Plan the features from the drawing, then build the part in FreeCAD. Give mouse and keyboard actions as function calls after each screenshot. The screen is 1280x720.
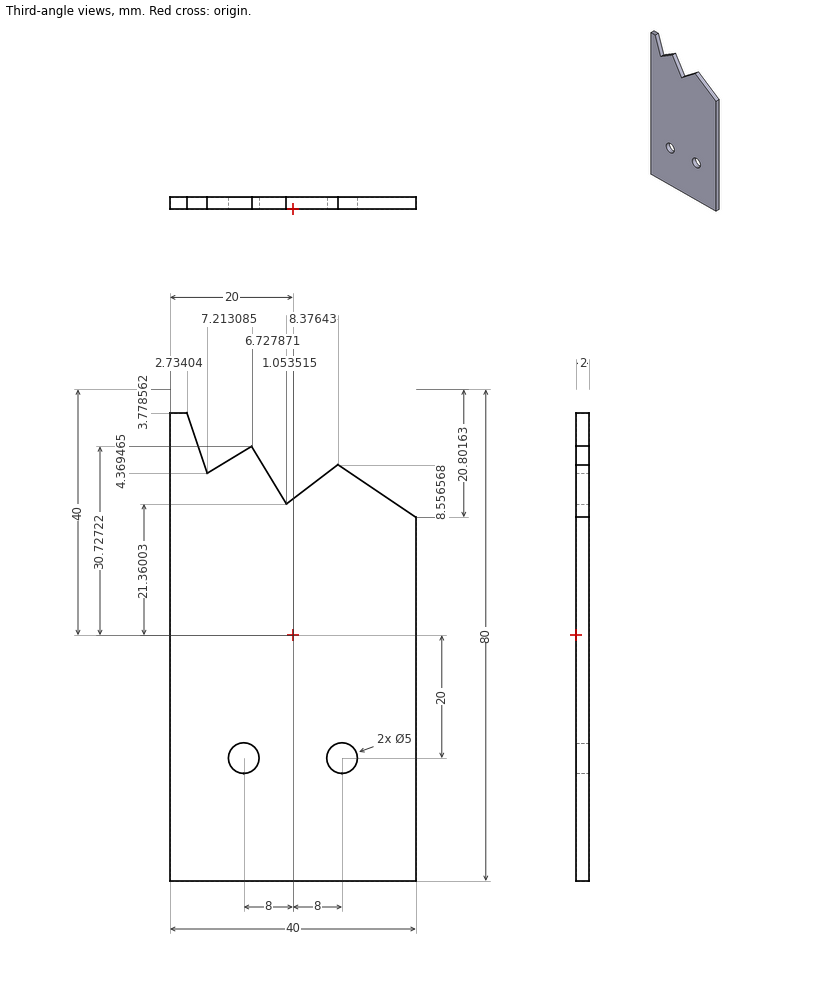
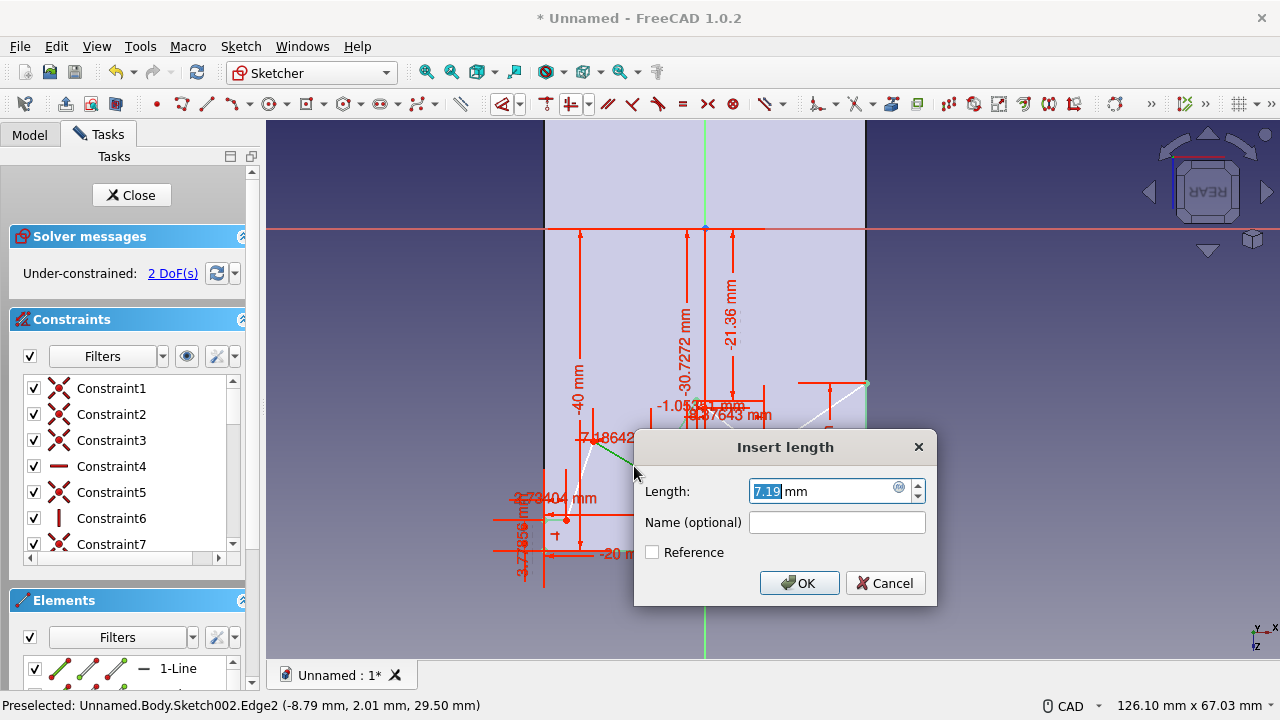
text(7.213085)
key(Return)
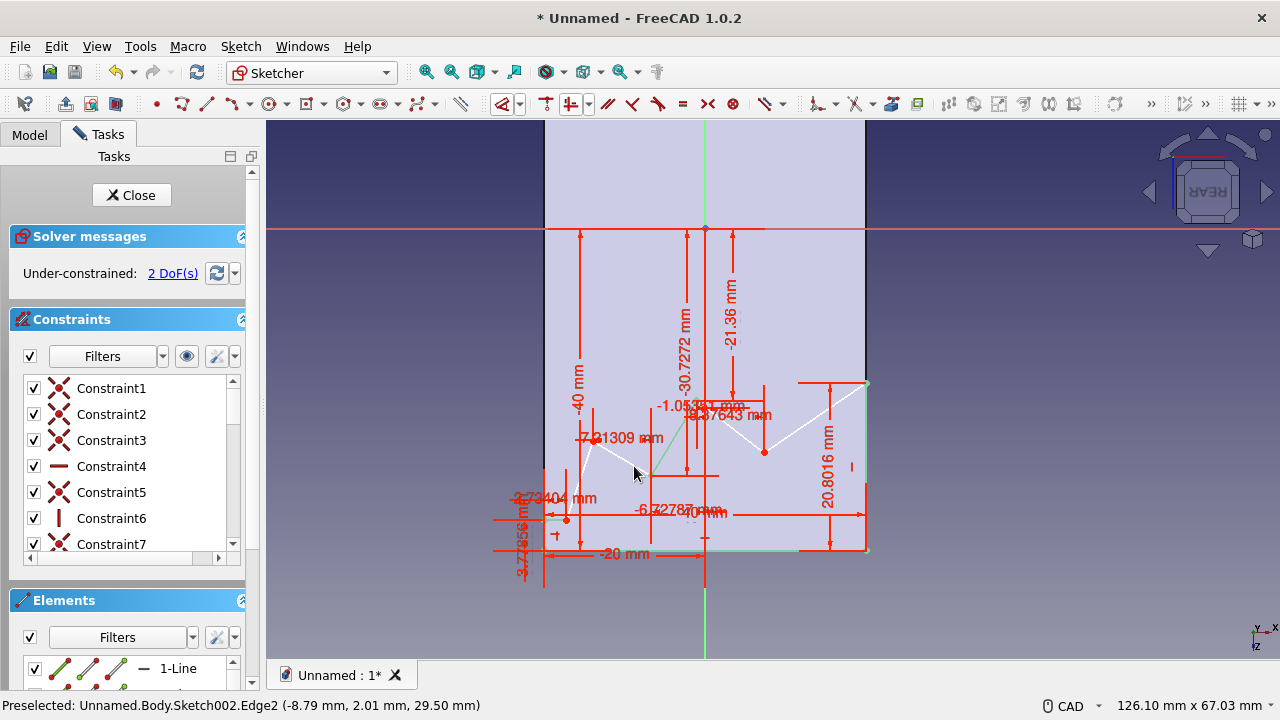
click(634, 466)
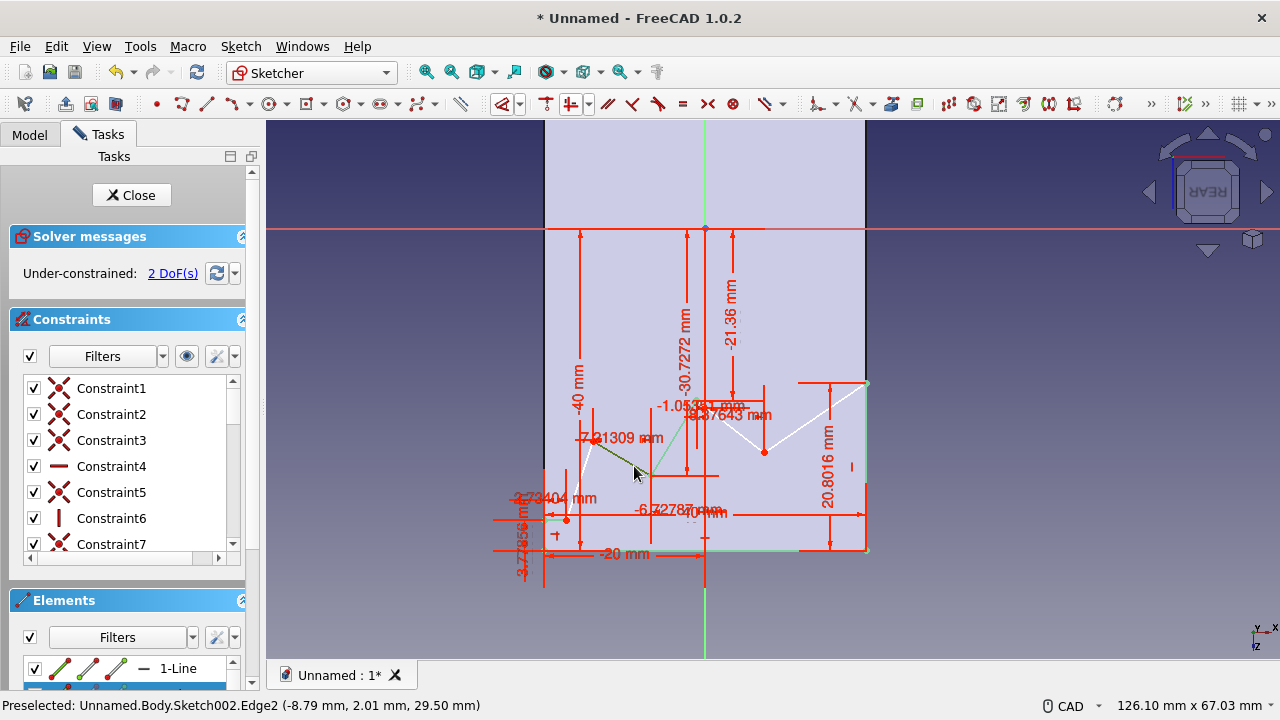
key(i)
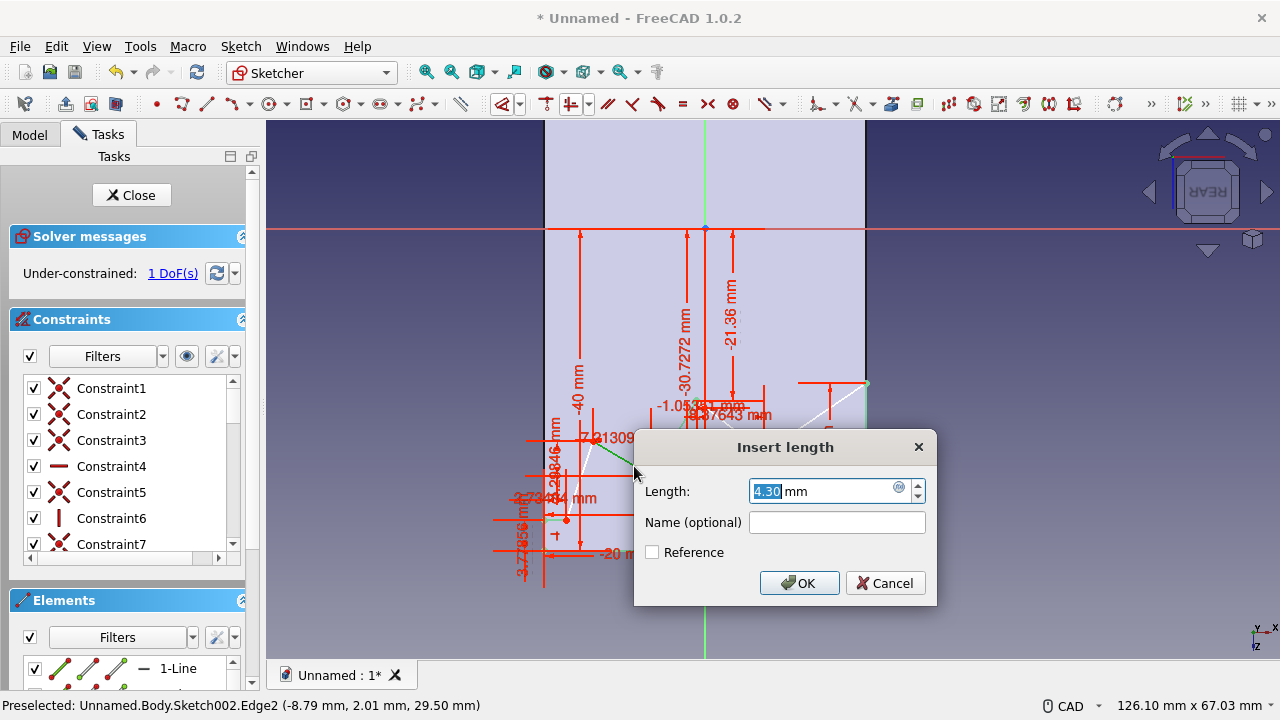
text(4.369465)
key(Return)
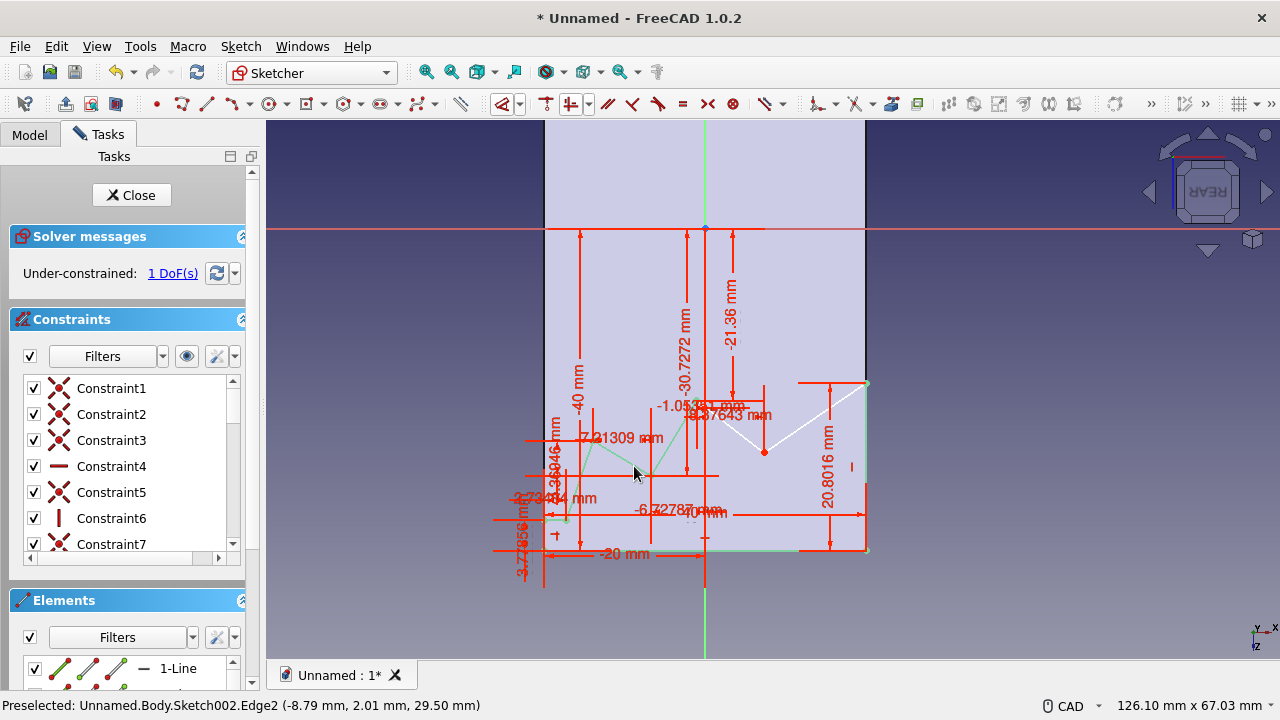
click(835, 404)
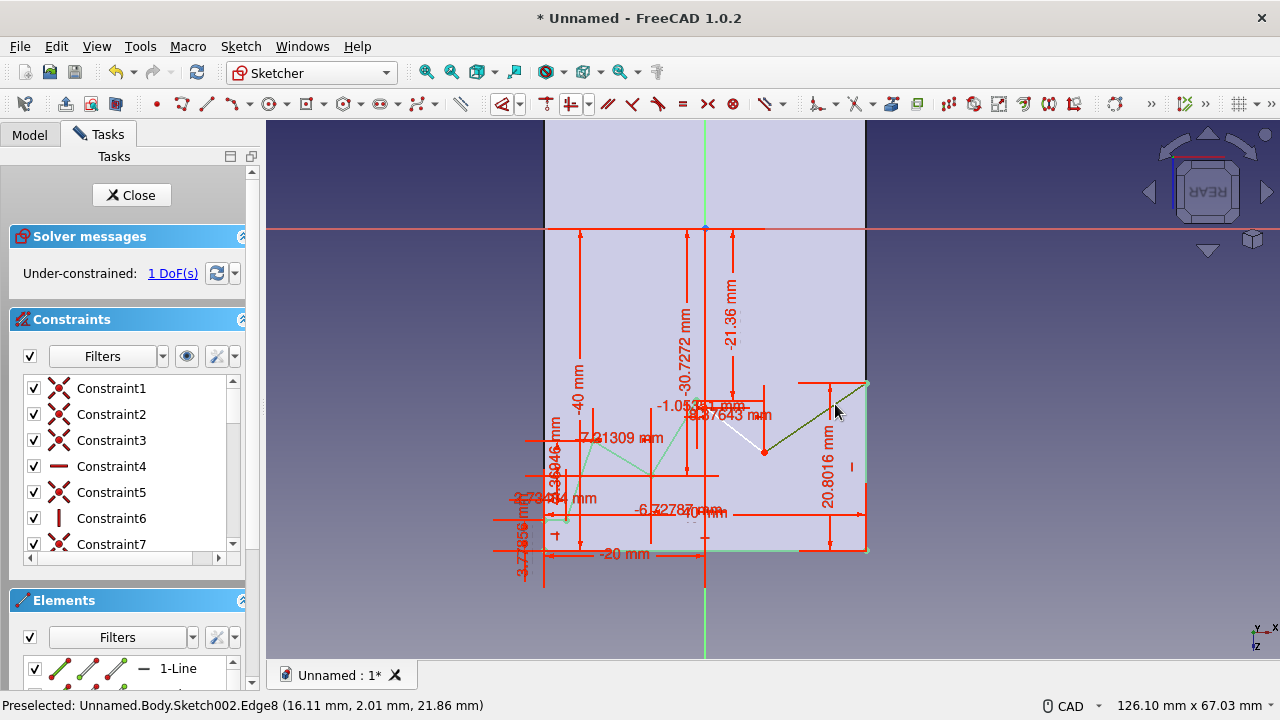
key(i)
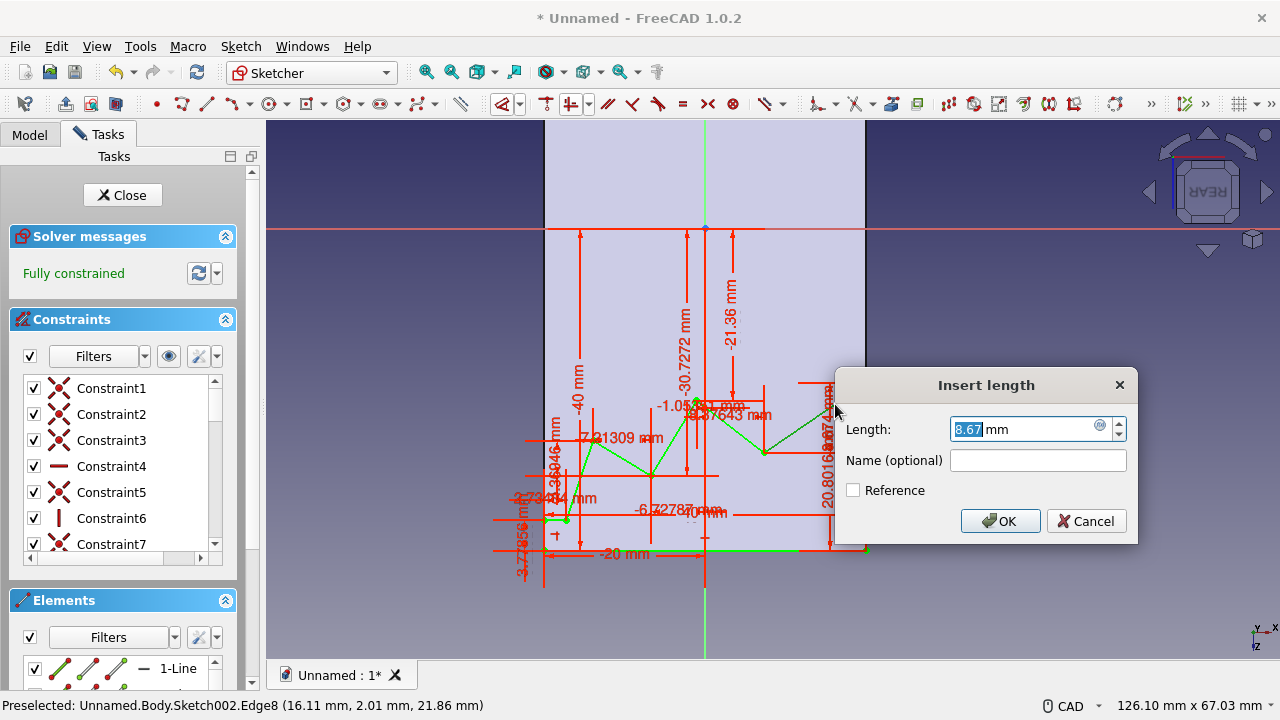
text(8.556568)
key(Return)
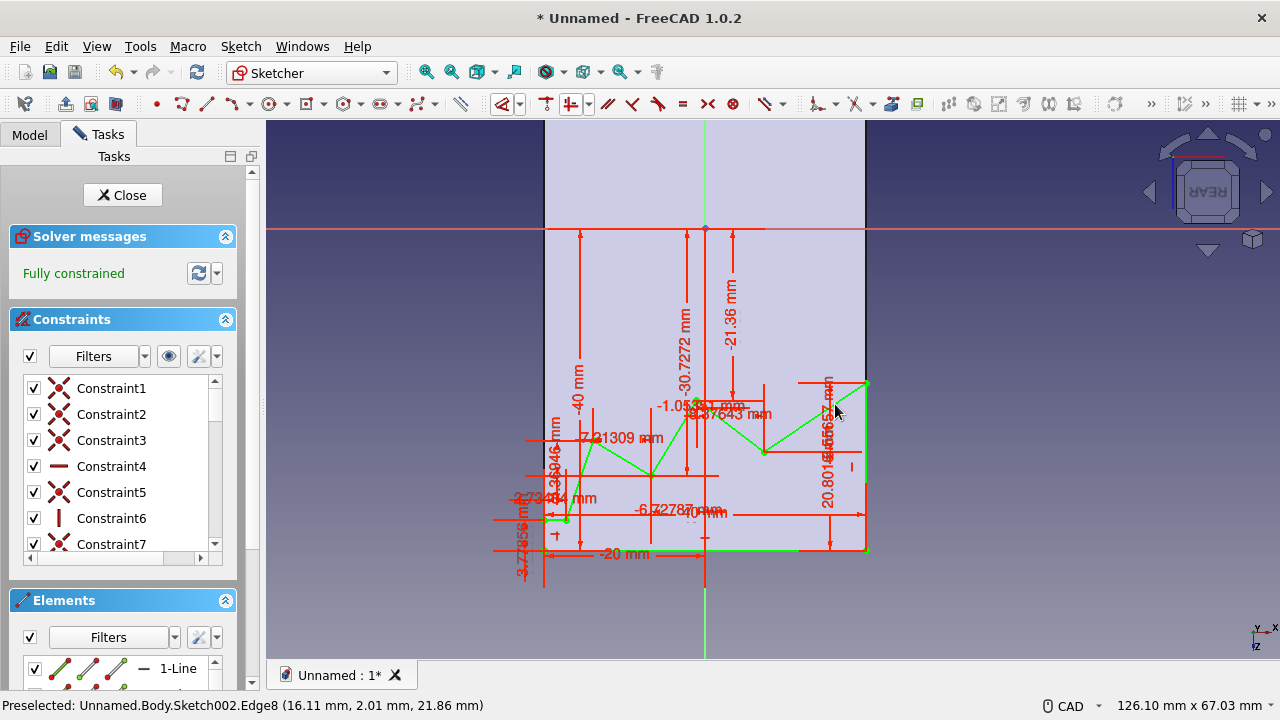
click(123, 195)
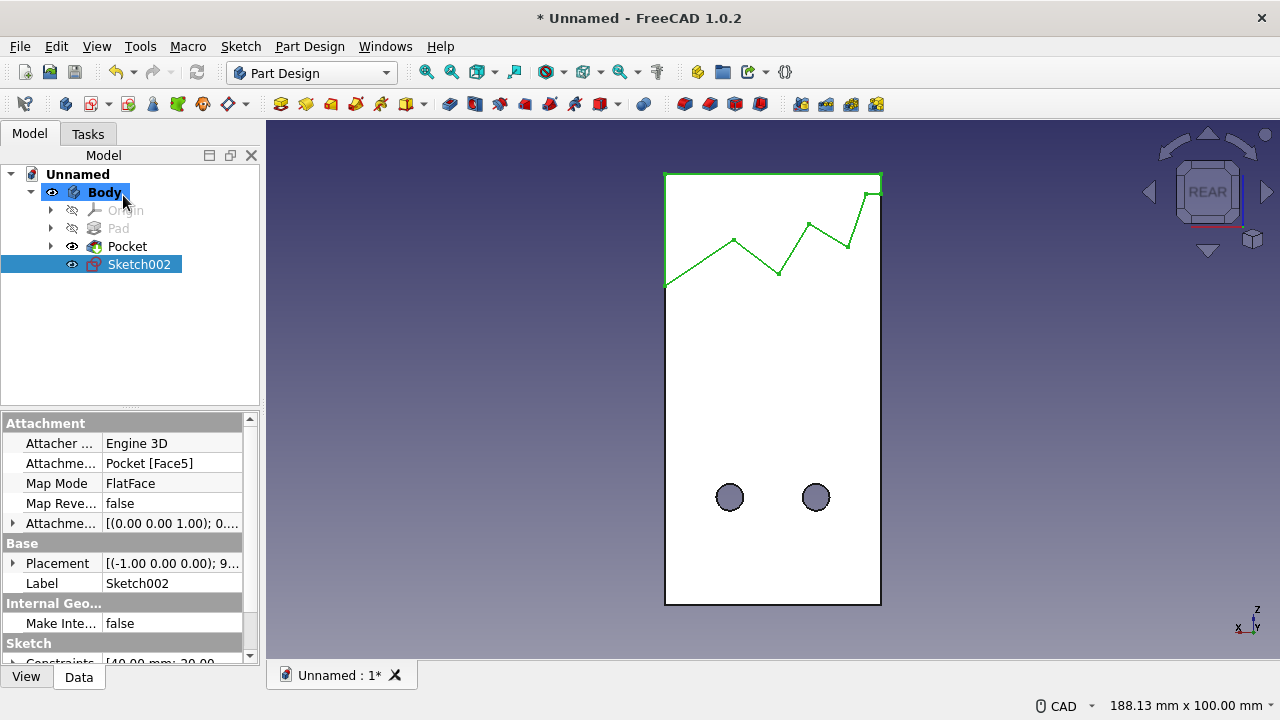
click(450, 104)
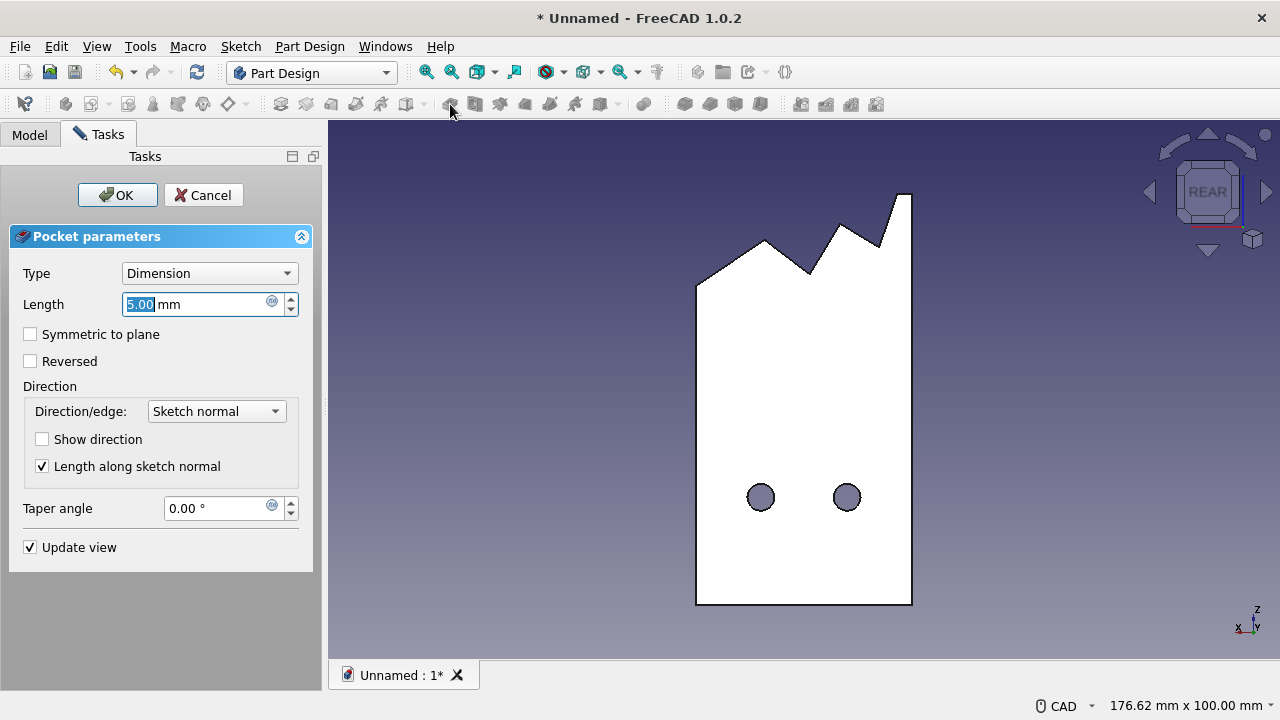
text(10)
key(Tab)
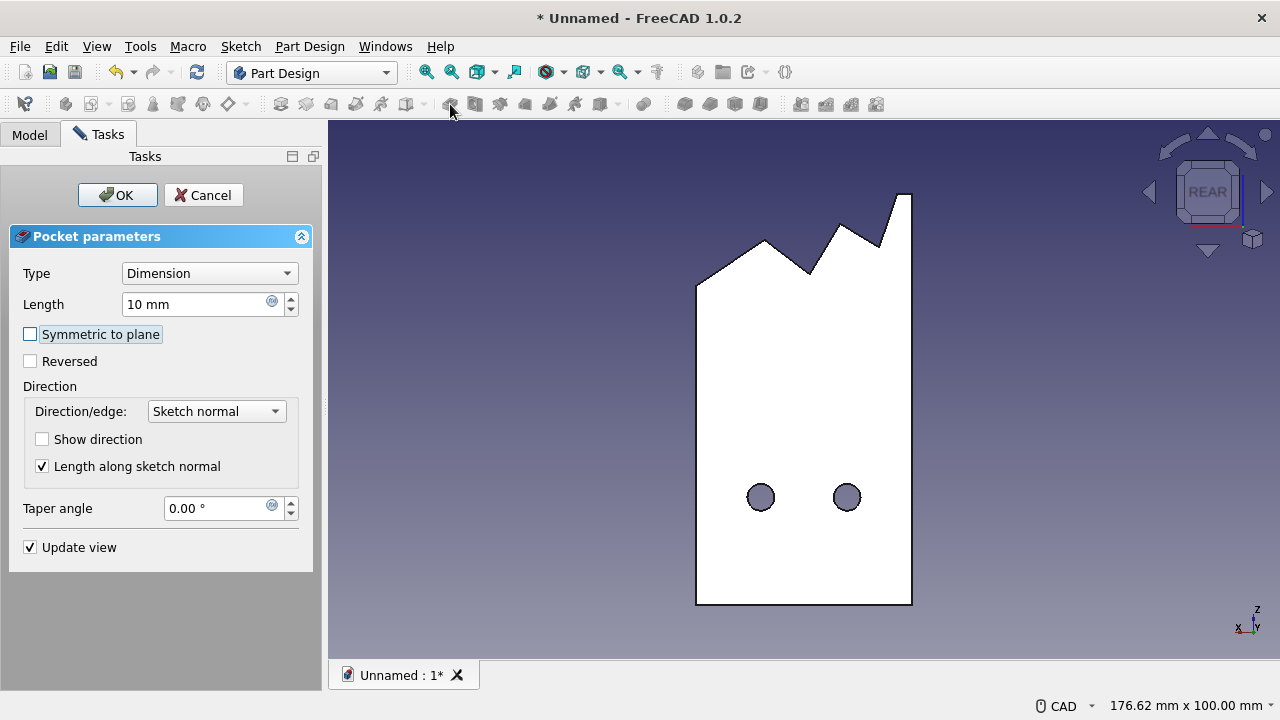
click(118, 195)